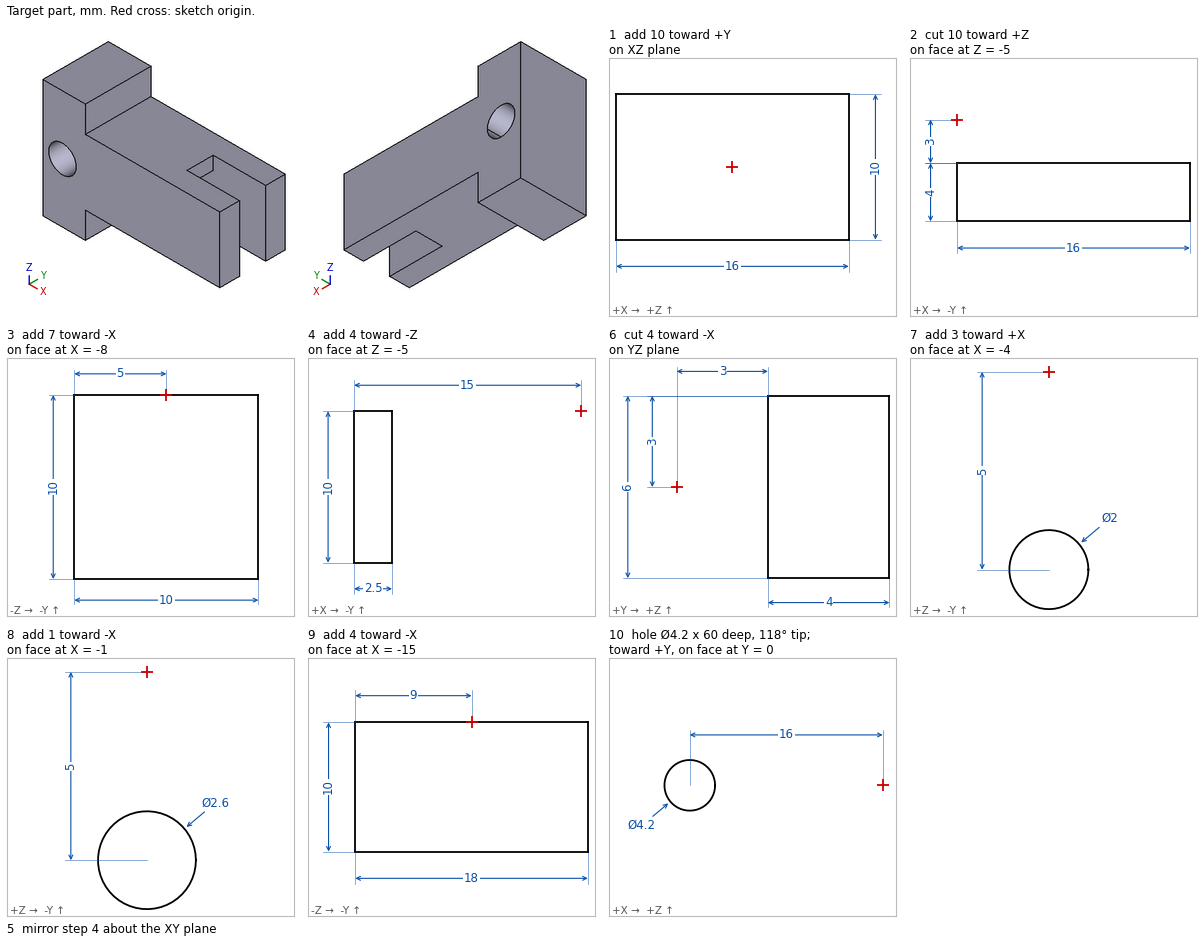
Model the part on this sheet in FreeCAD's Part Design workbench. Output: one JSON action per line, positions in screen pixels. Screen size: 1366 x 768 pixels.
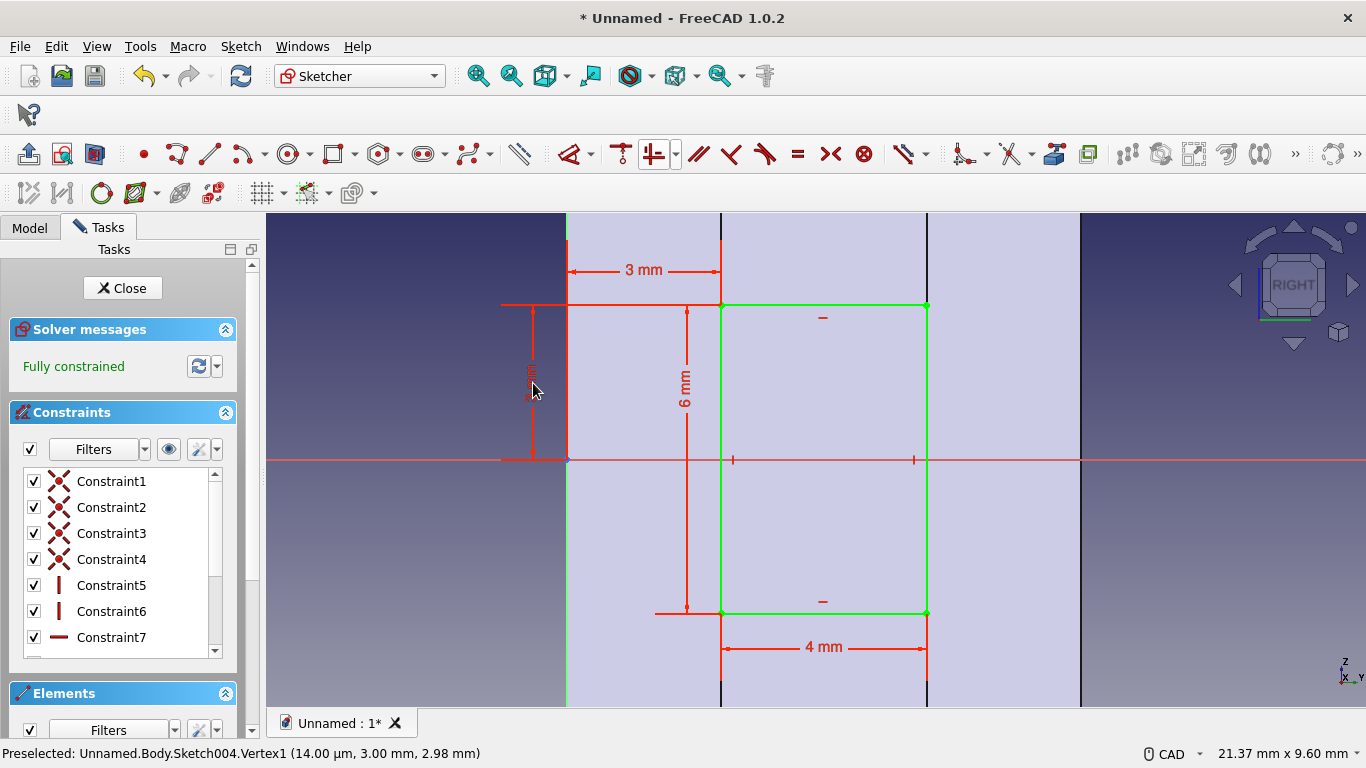
{"action": "left_click", "coordinate": [123, 288]}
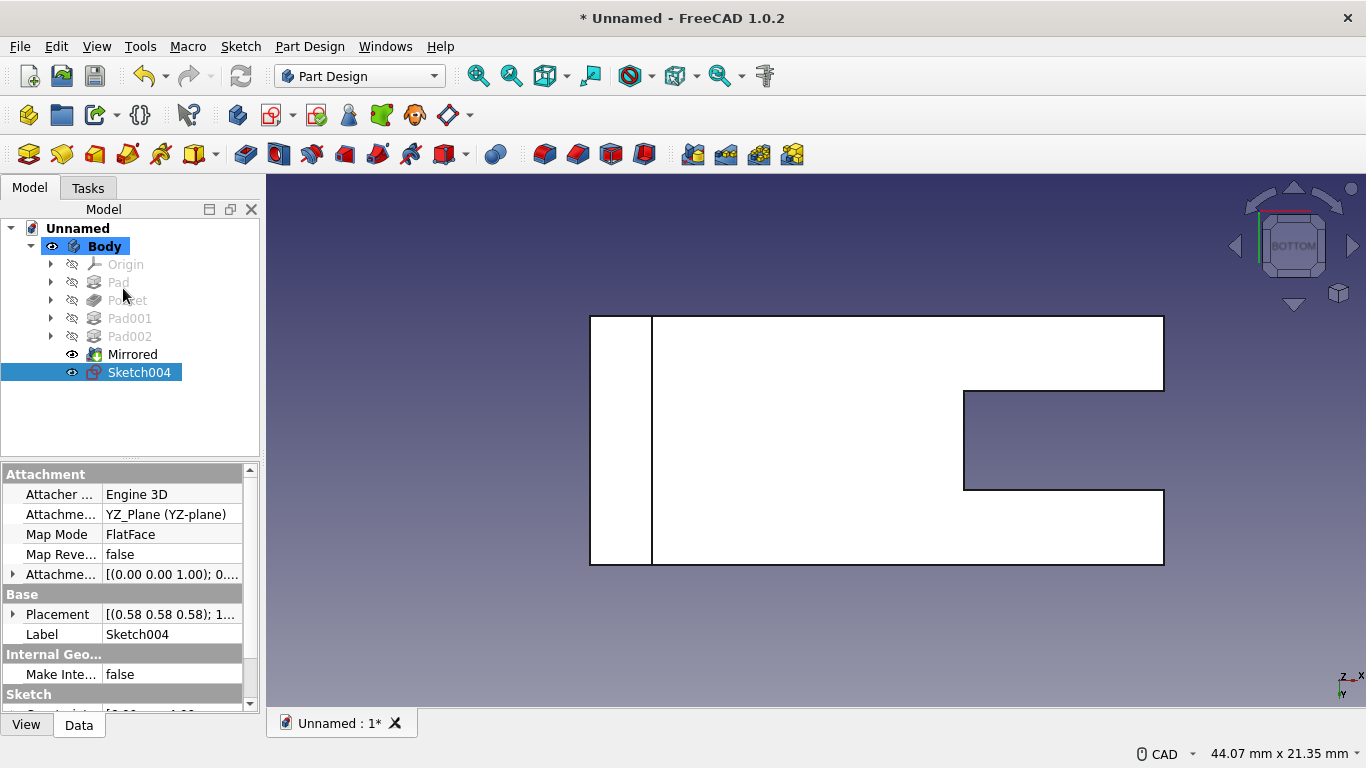
{"action": "left_click", "coordinate": [246, 154]}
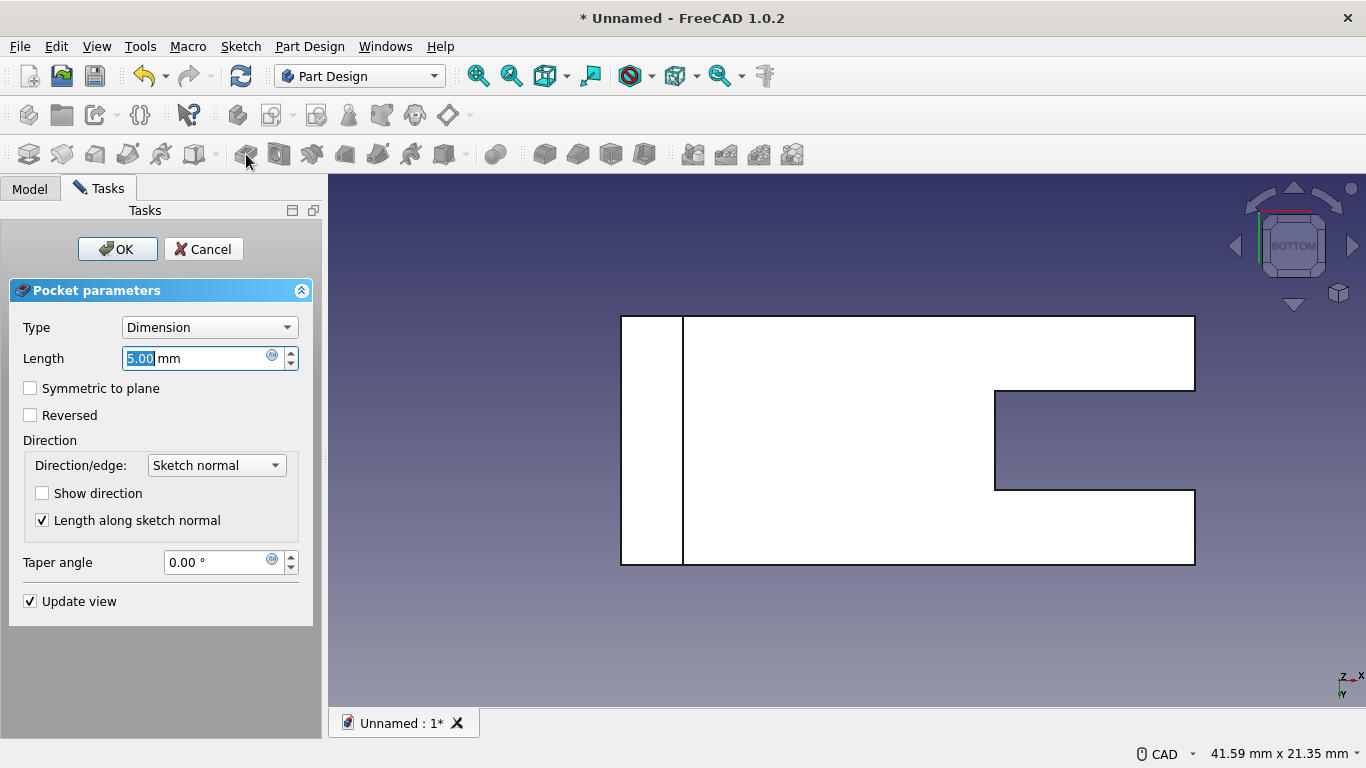
{"action": "type", "text": "4"}
{"action": "key", "text": "Tab"}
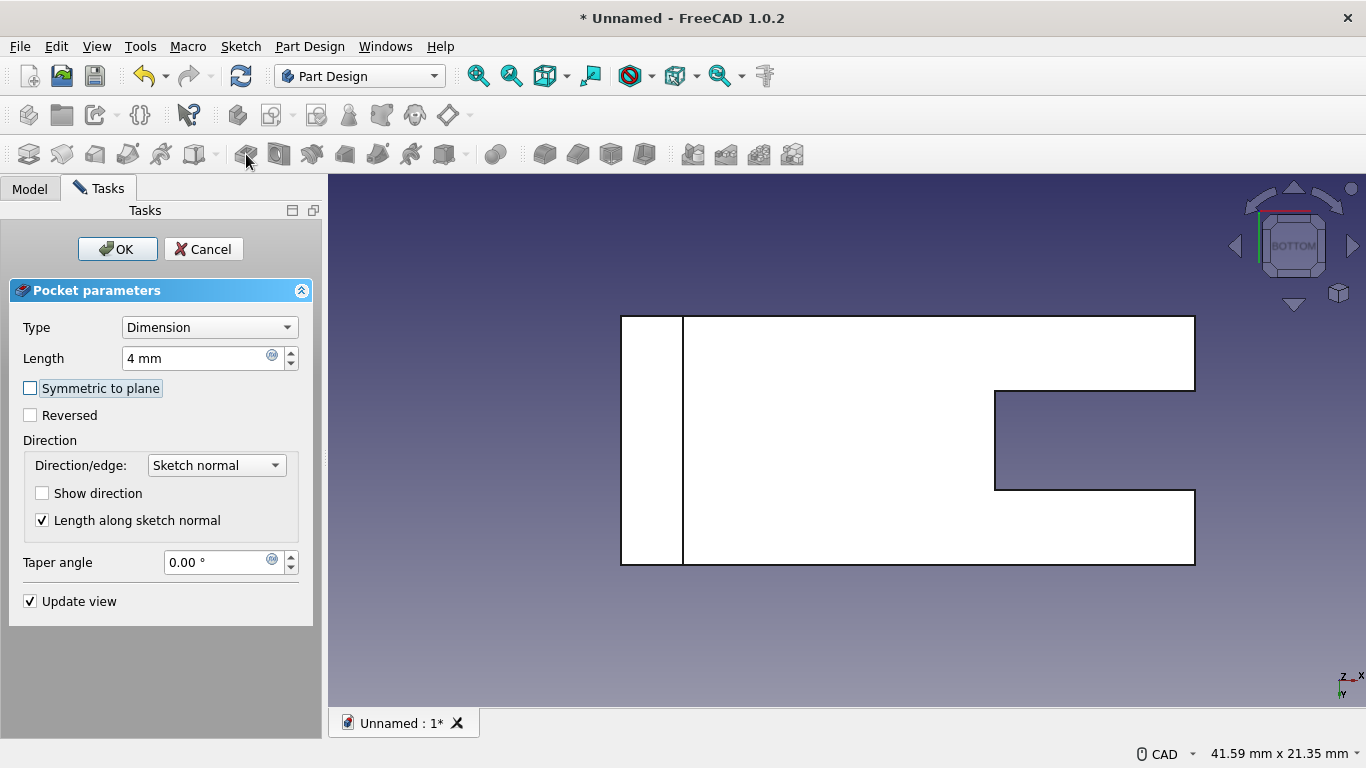
{"action": "left_click", "coordinate": [118, 249]}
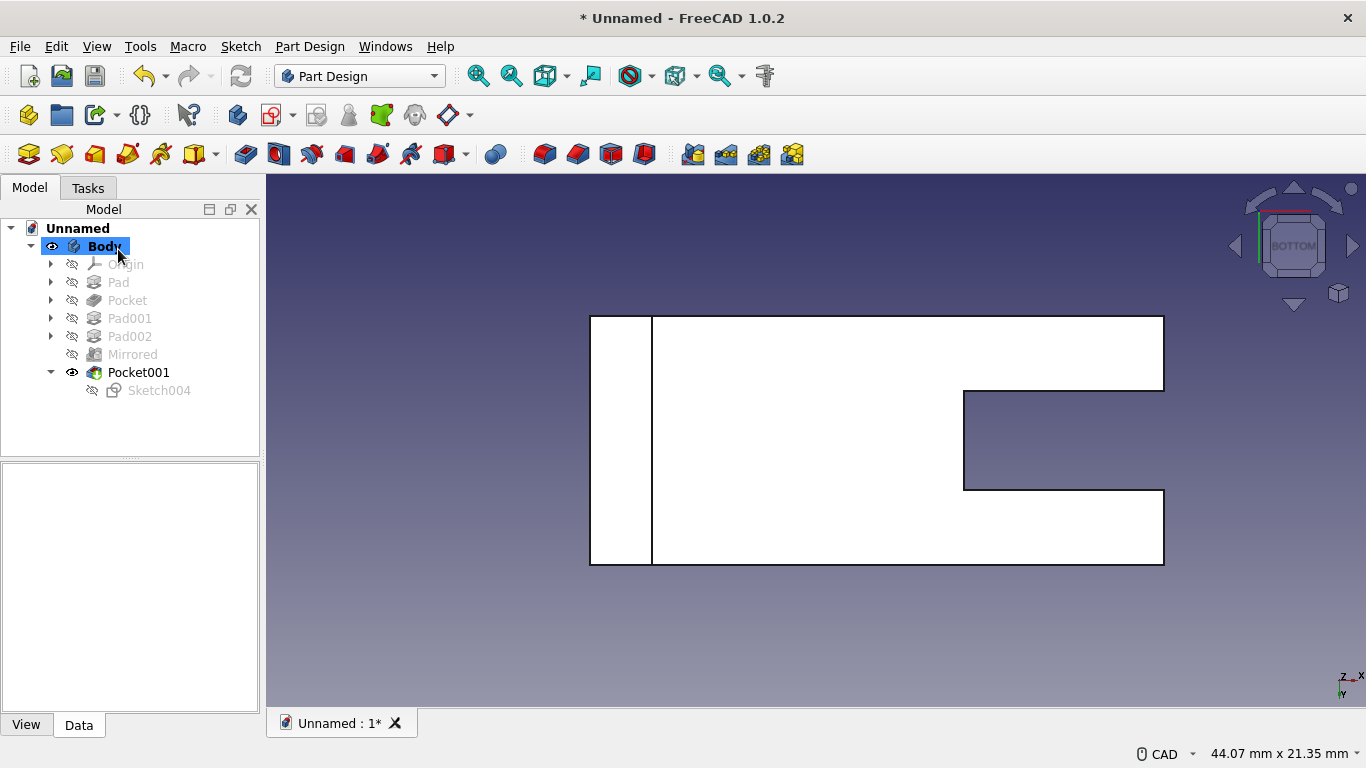
{"action": "key", "text": "0"}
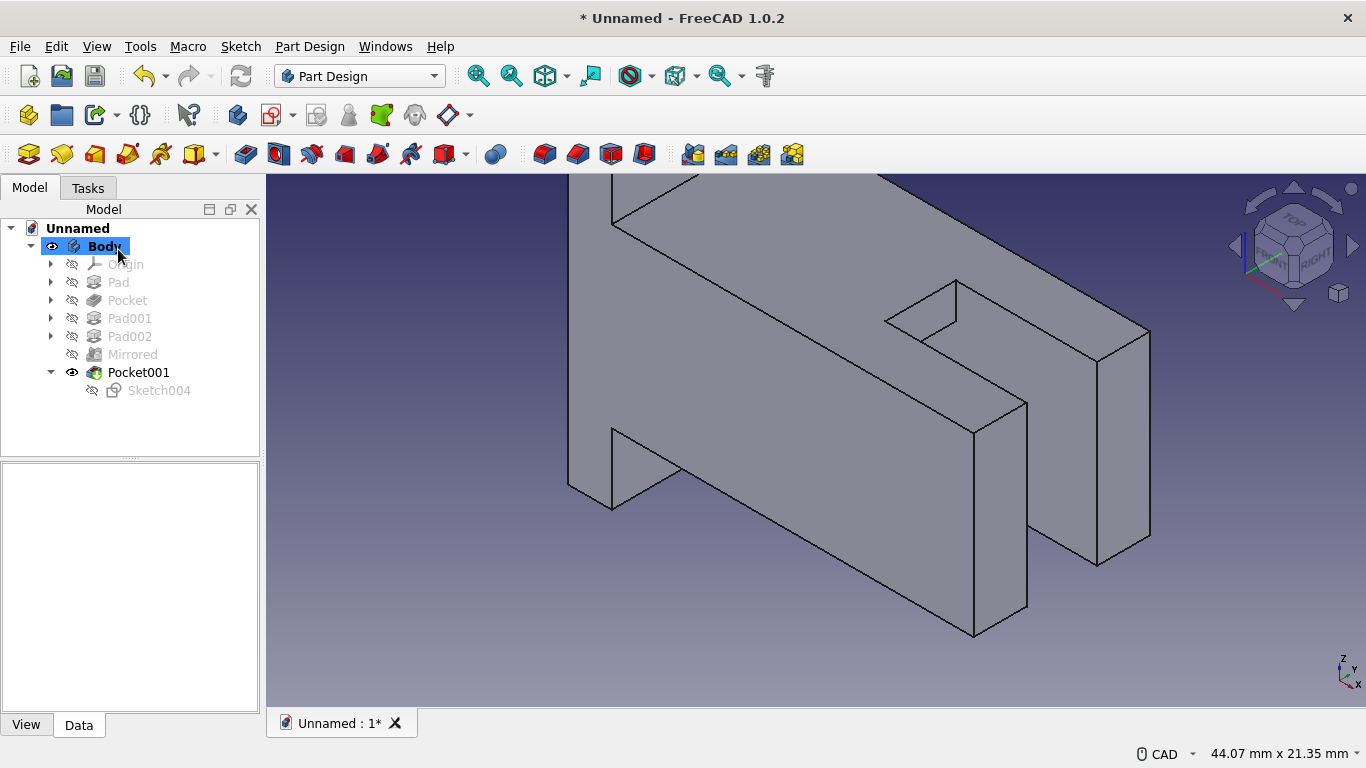
{"action": "left_click", "coordinate": [479, 76]}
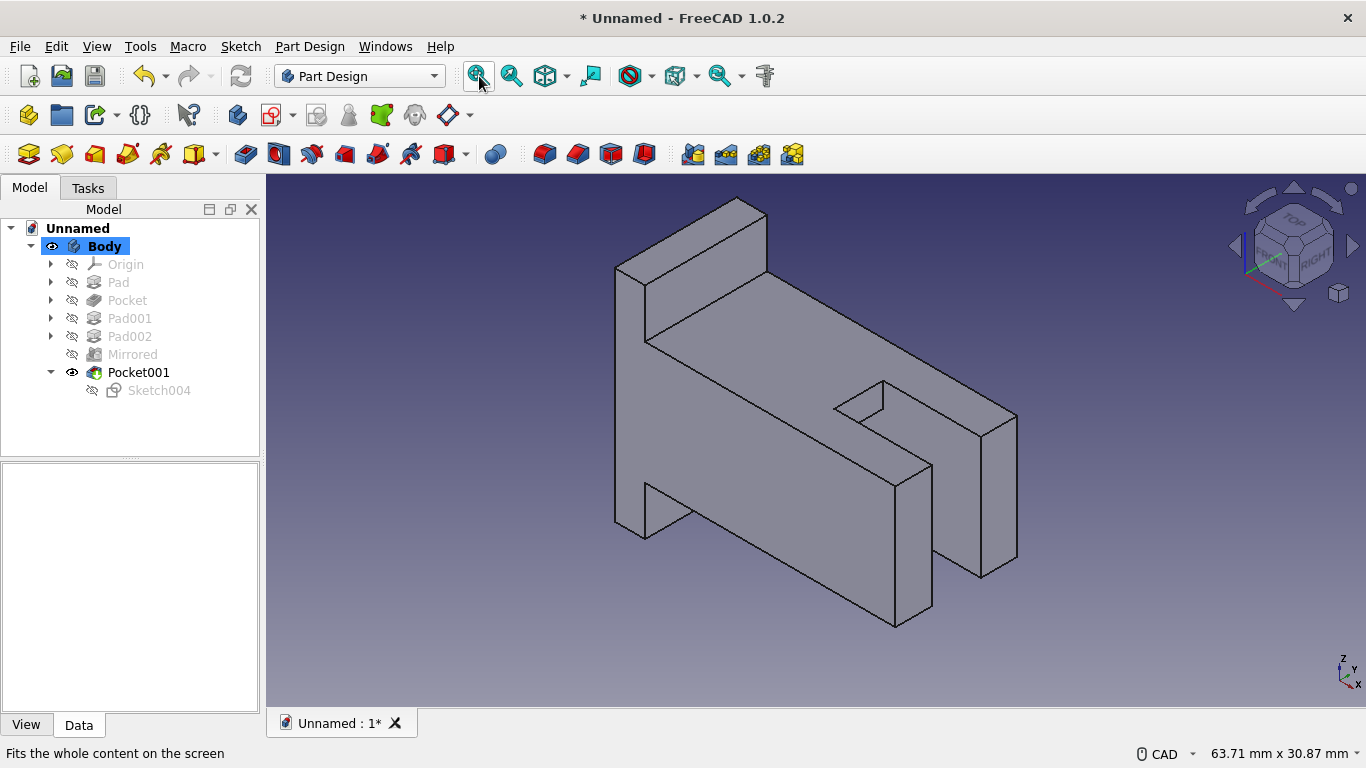
{"action": "key", "text": "3"}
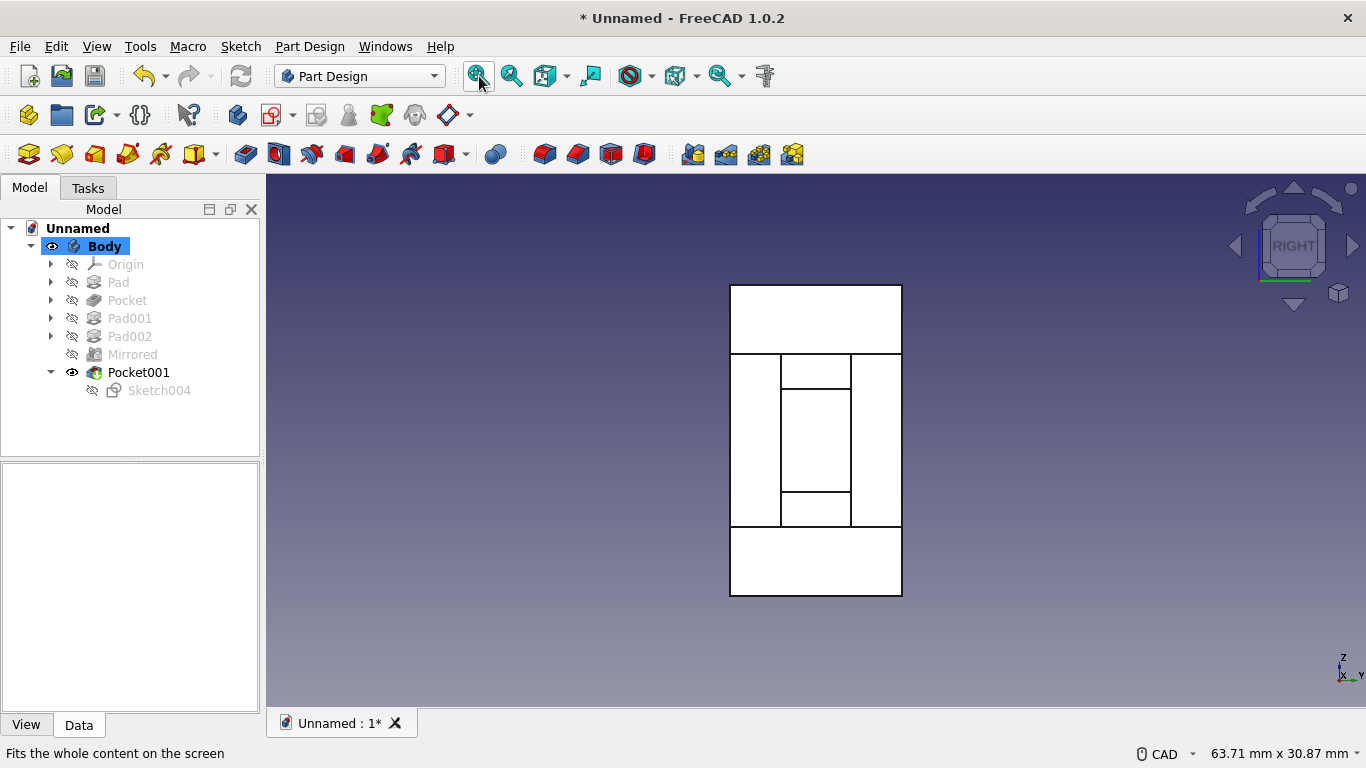
{"action": "left_click", "coordinate": [816, 425]}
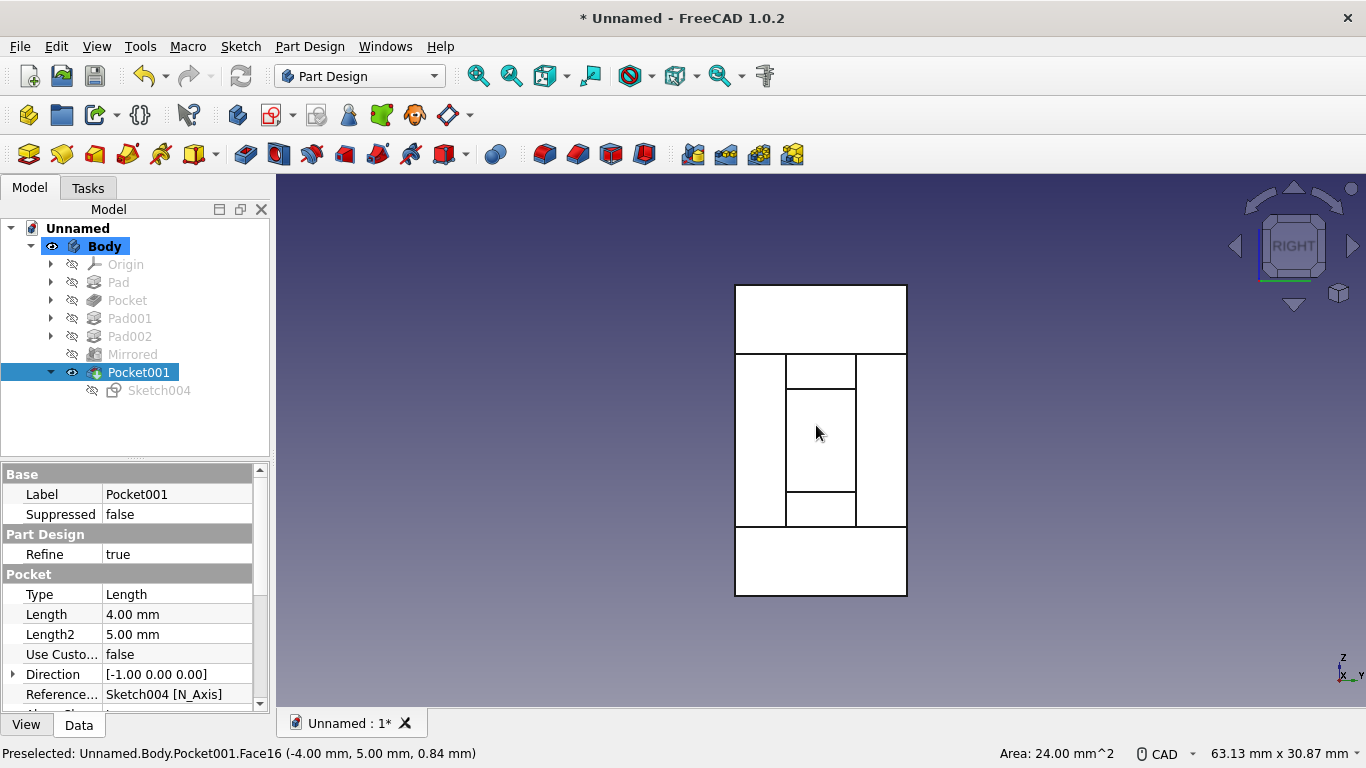
{"action": "left_click", "coordinate": [270, 116]}